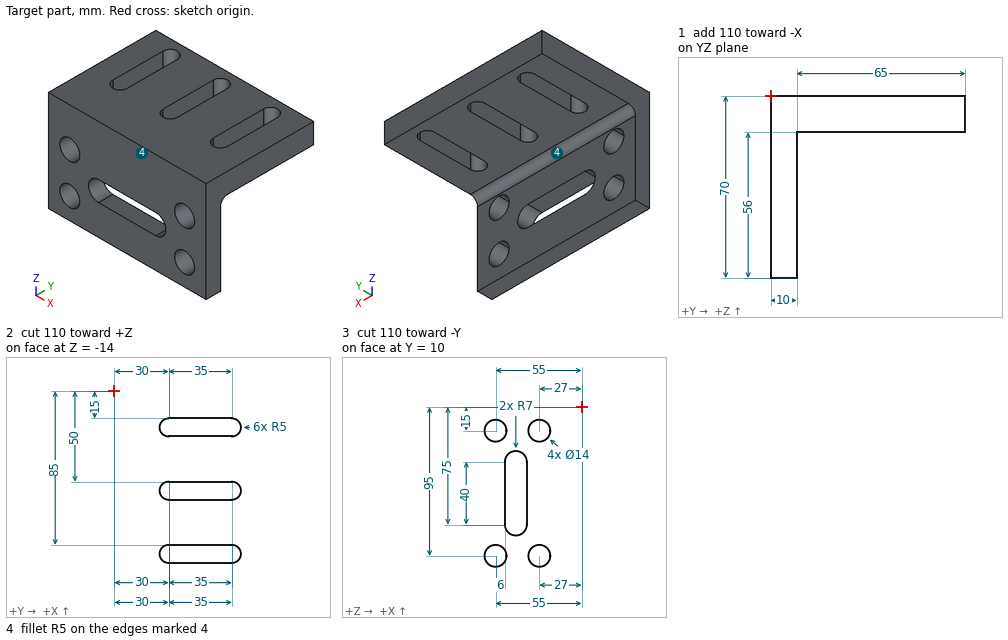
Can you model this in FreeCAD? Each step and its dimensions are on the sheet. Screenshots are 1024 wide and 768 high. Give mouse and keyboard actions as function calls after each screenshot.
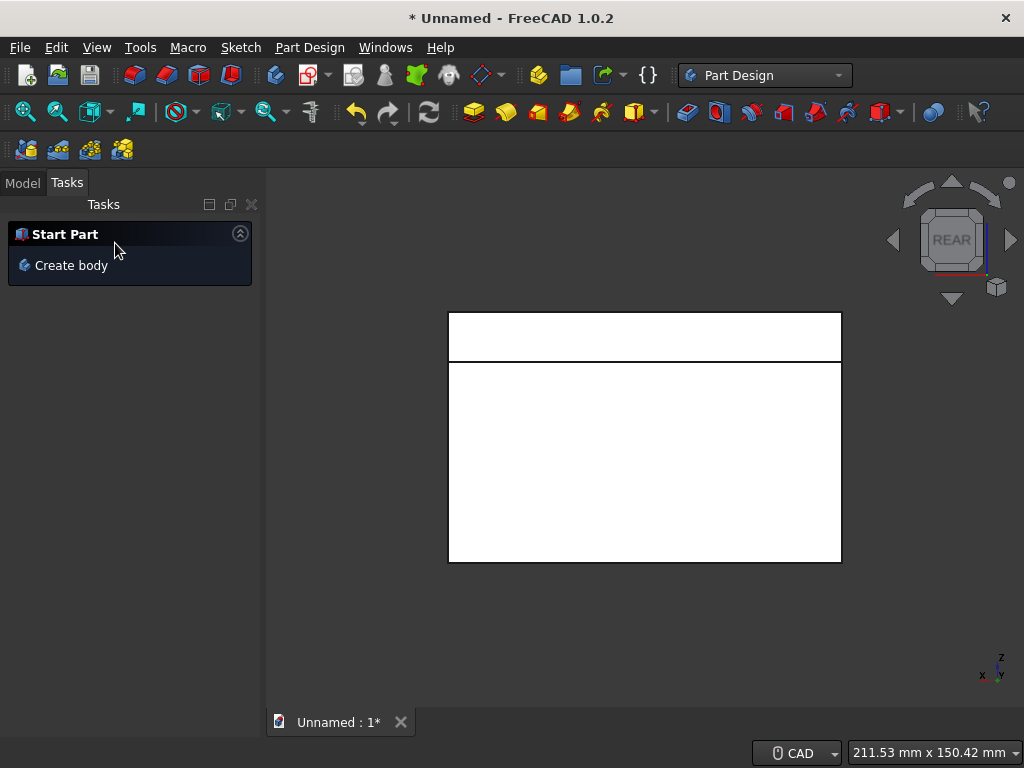
click(645, 462)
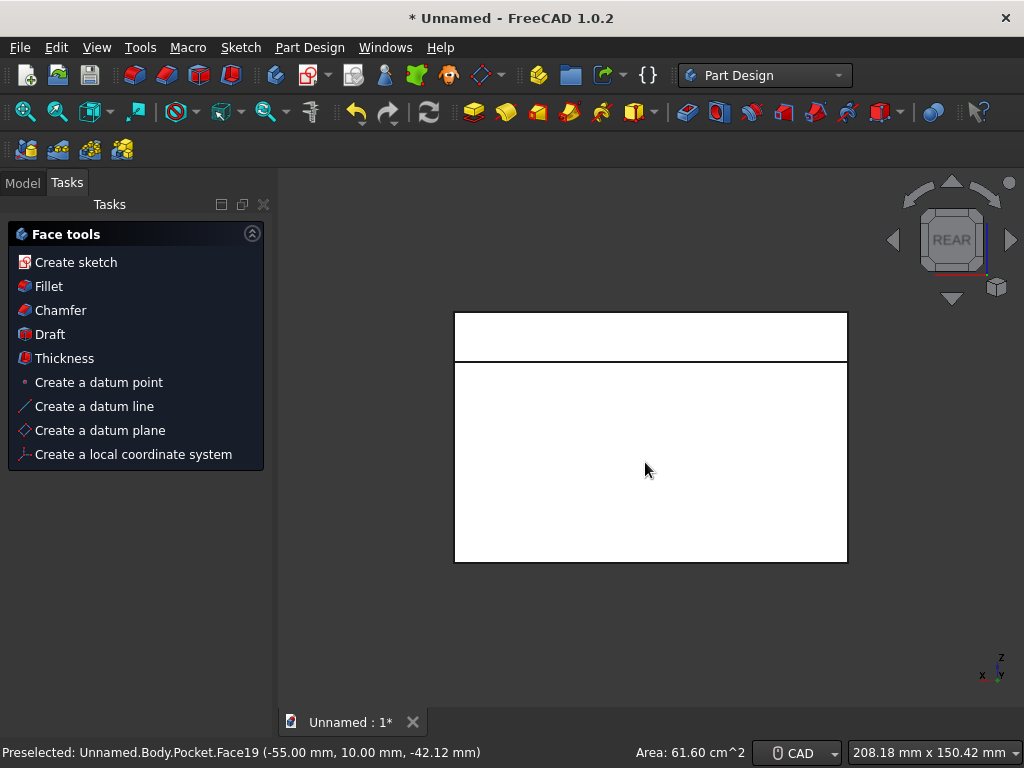
click(308, 76)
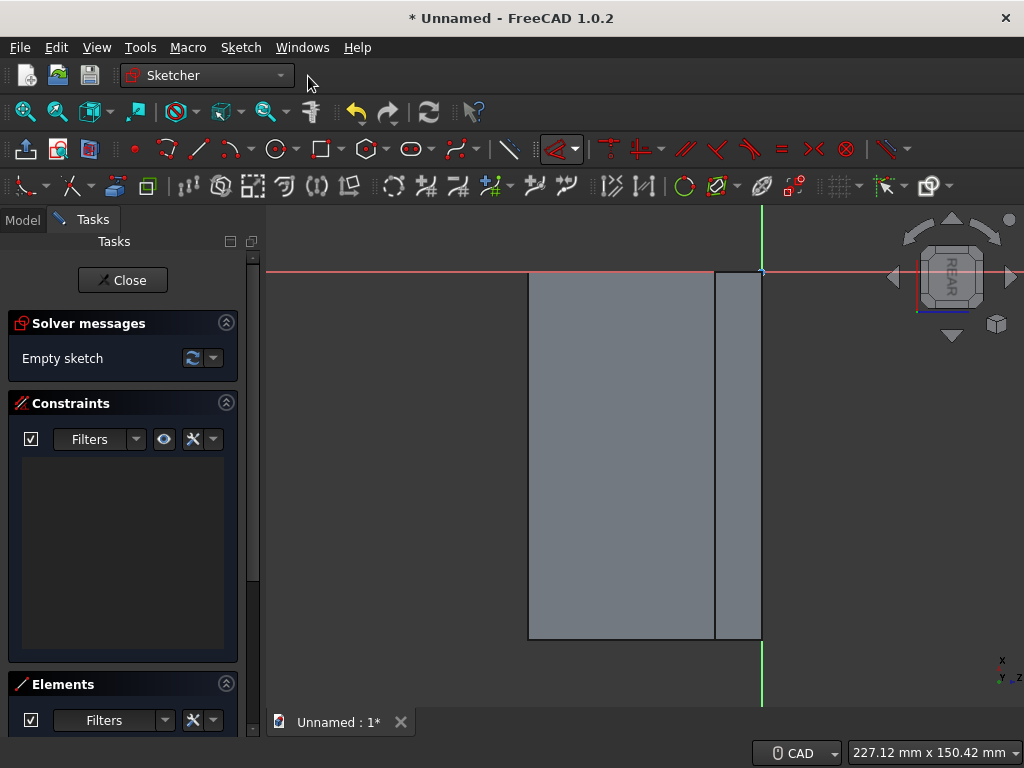
key(q)
key(s)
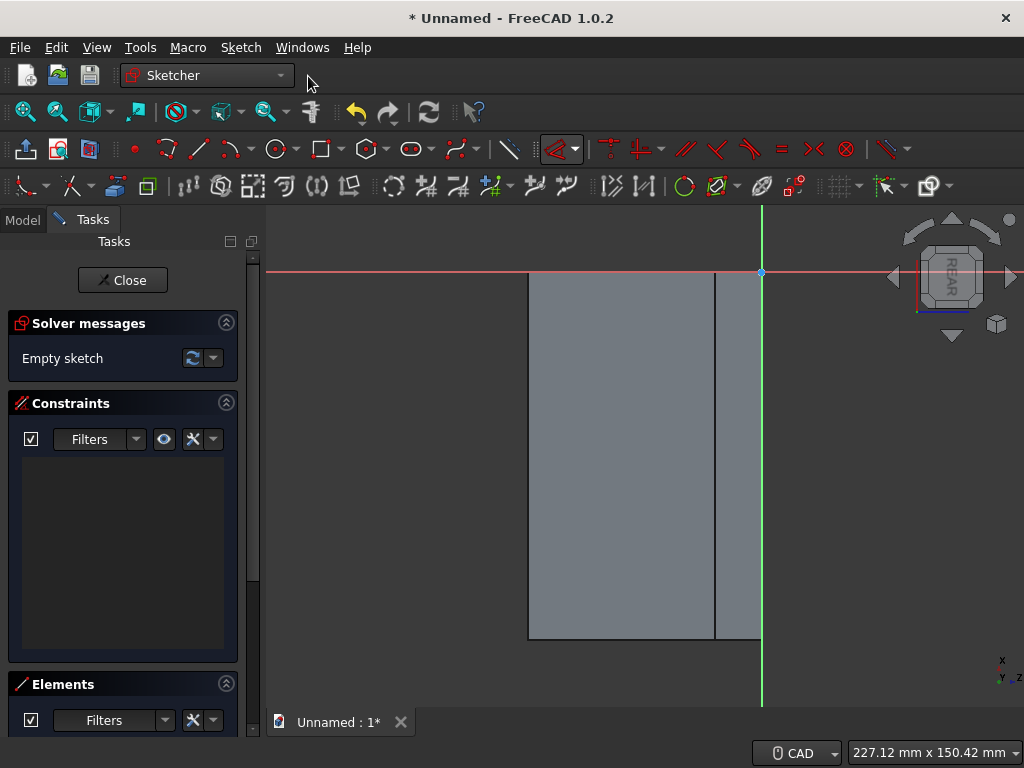
click(412, 150)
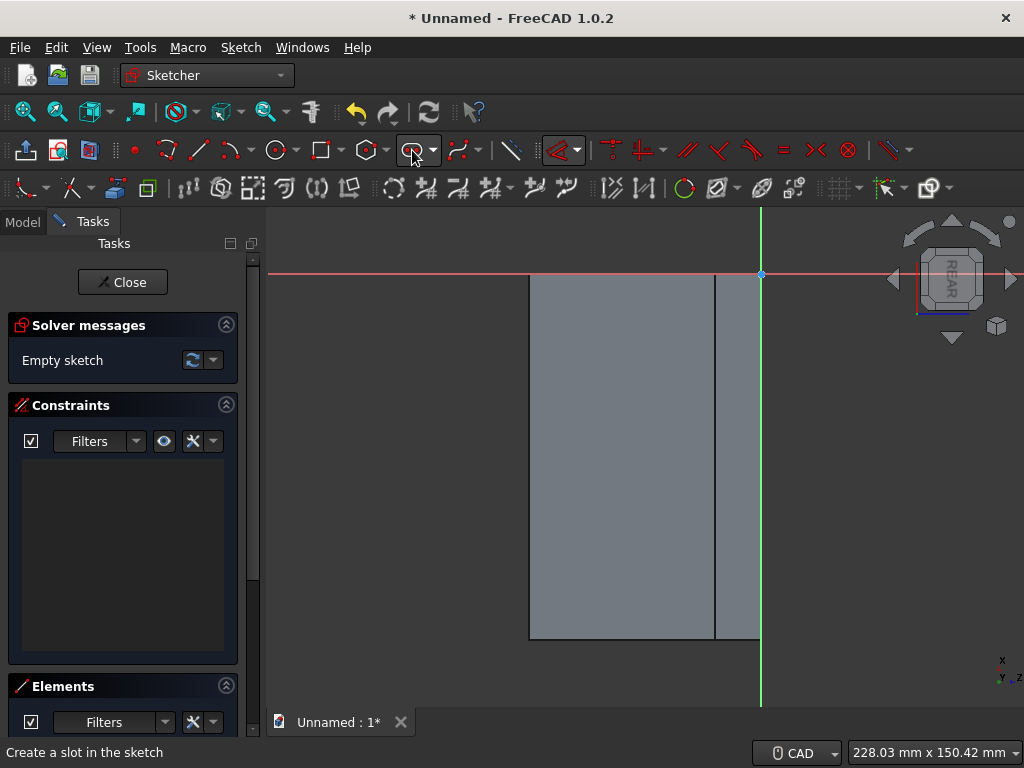
click(622, 523)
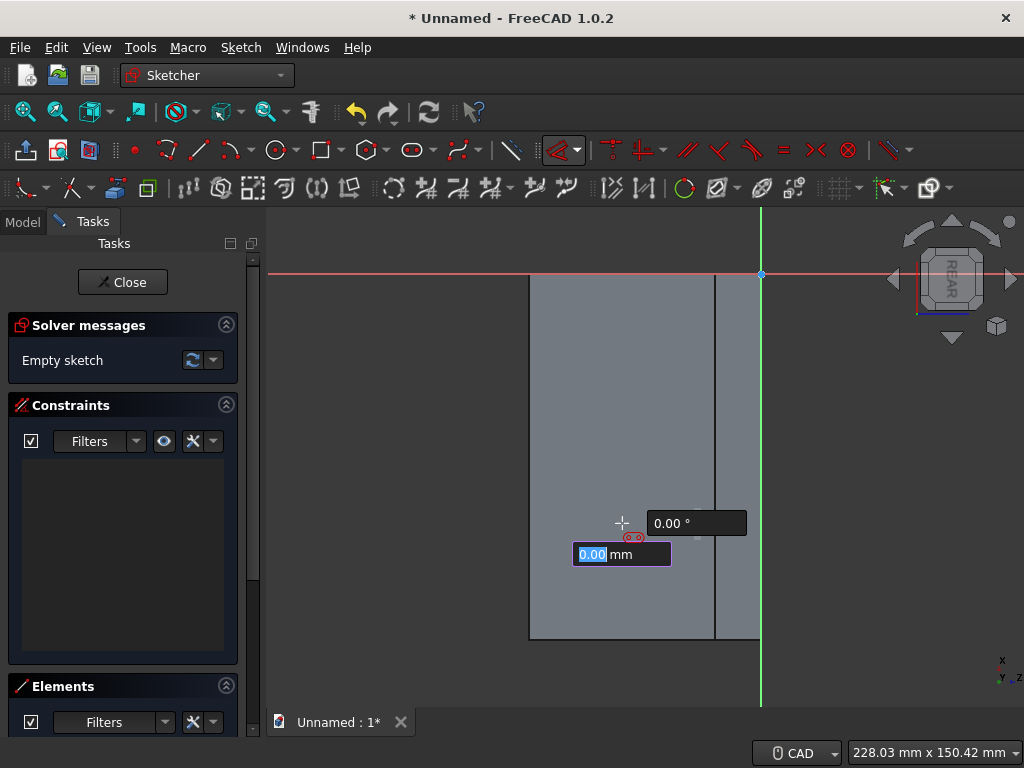
click(622, 391)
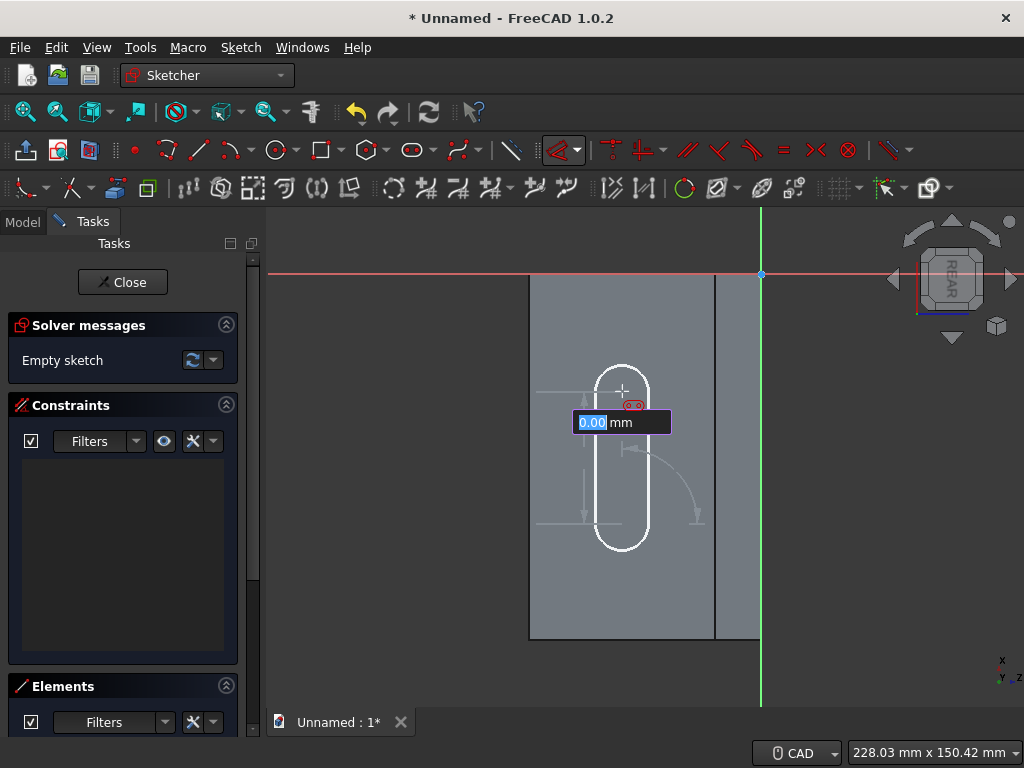
click(598, 457)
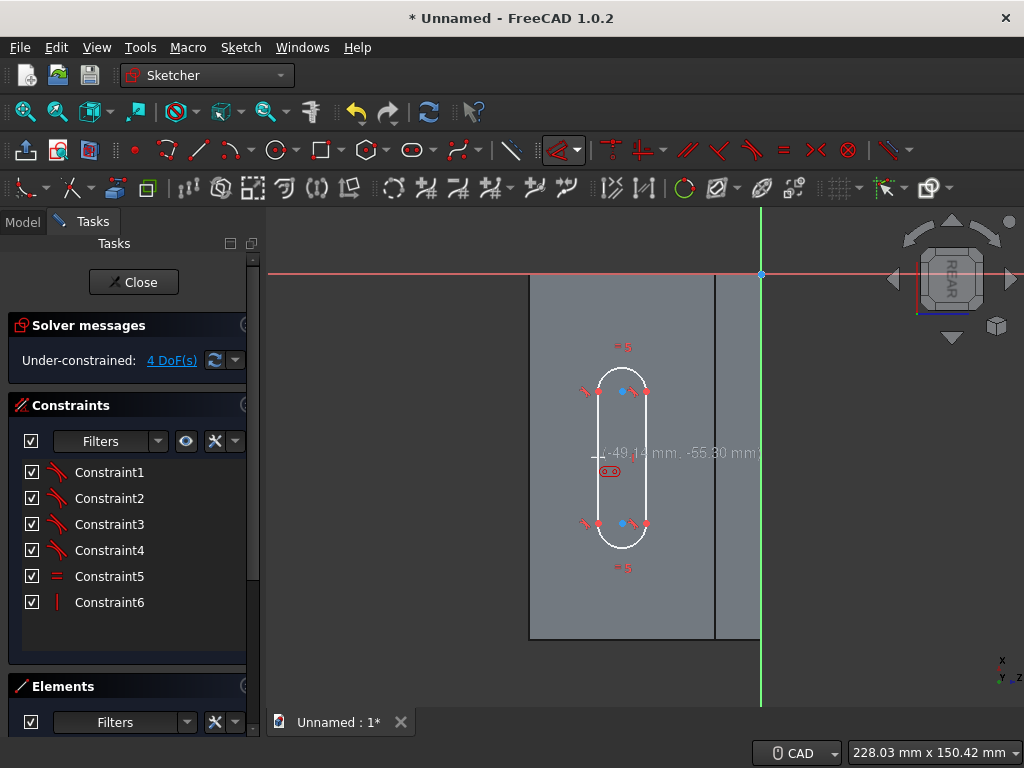
key(g)
key(c)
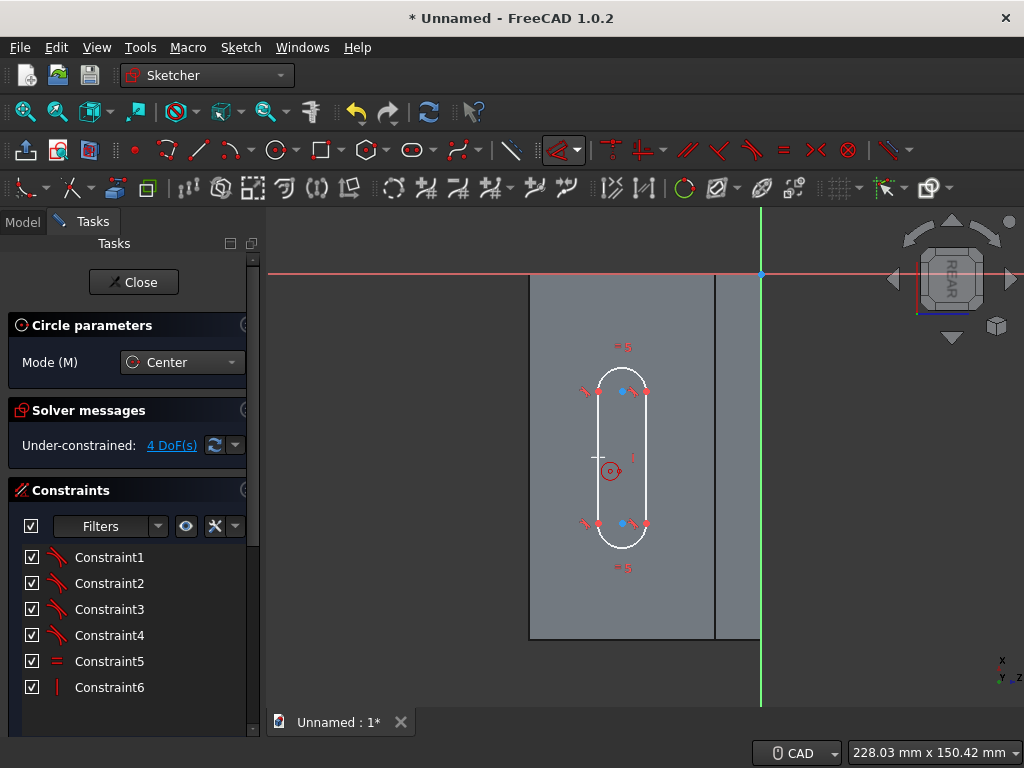
click(579, 590)
move(595, 574)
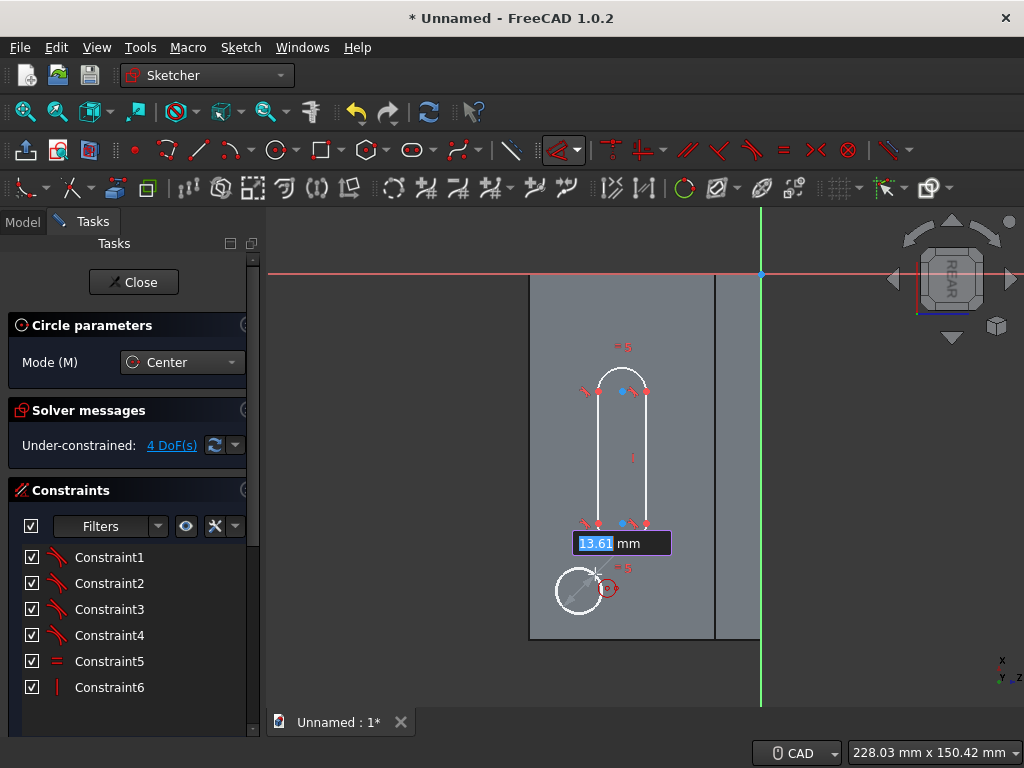
text(14)
key(Return)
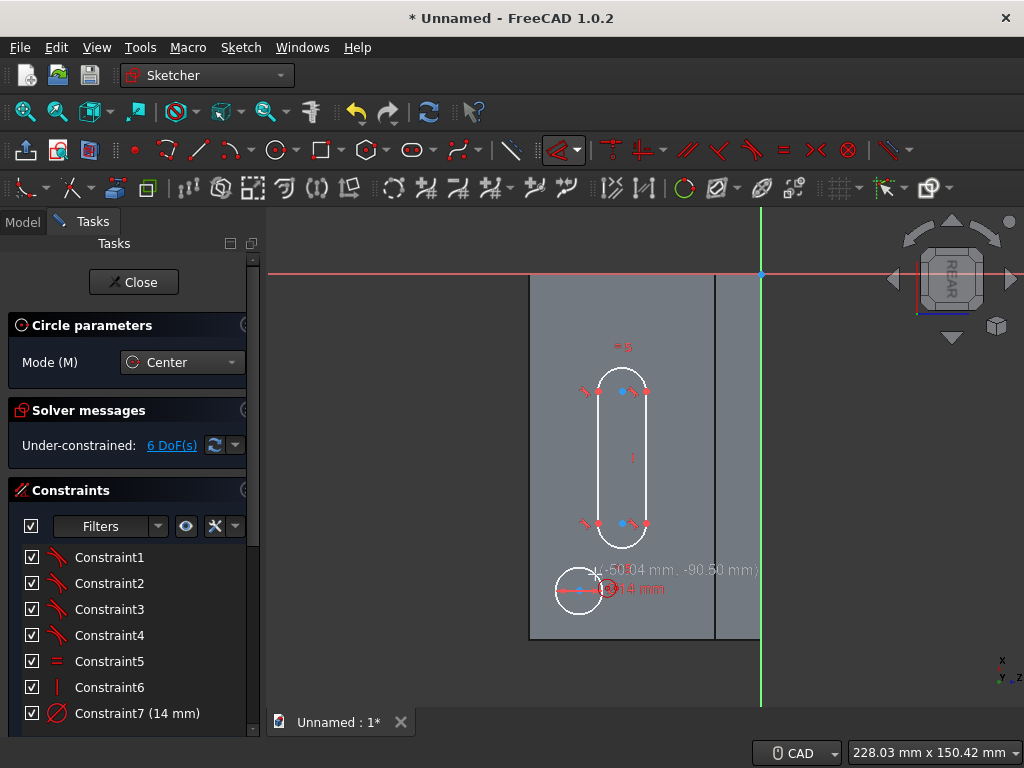
click(579, 324)
move(595, 308)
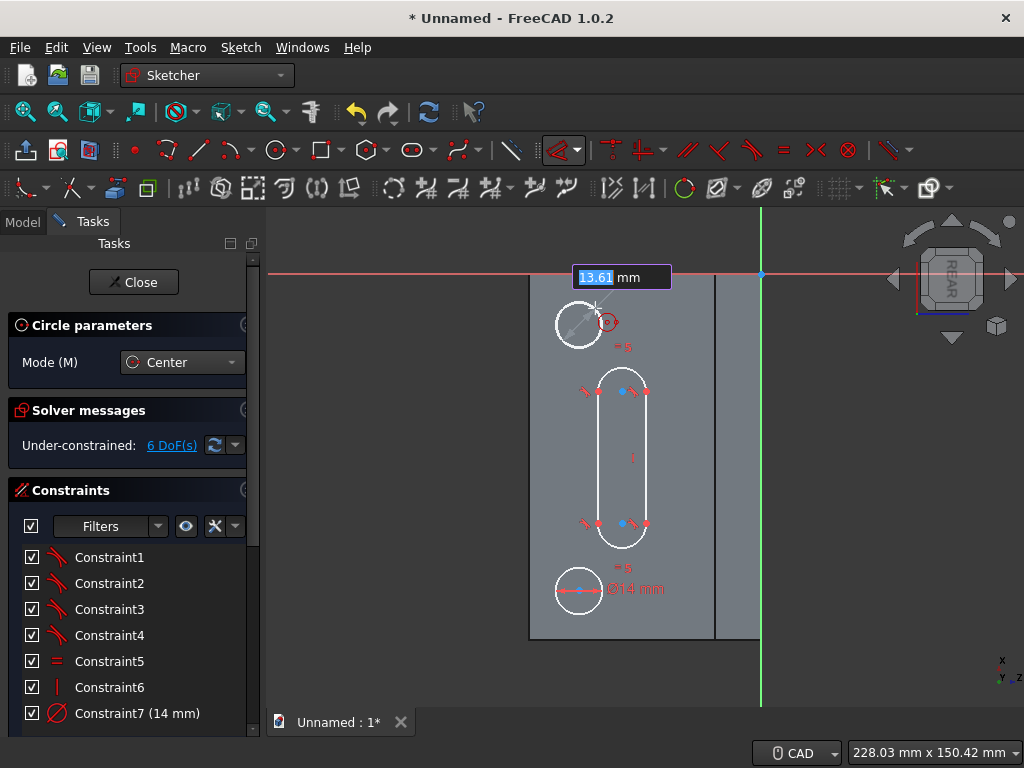
text(14)
key(Return)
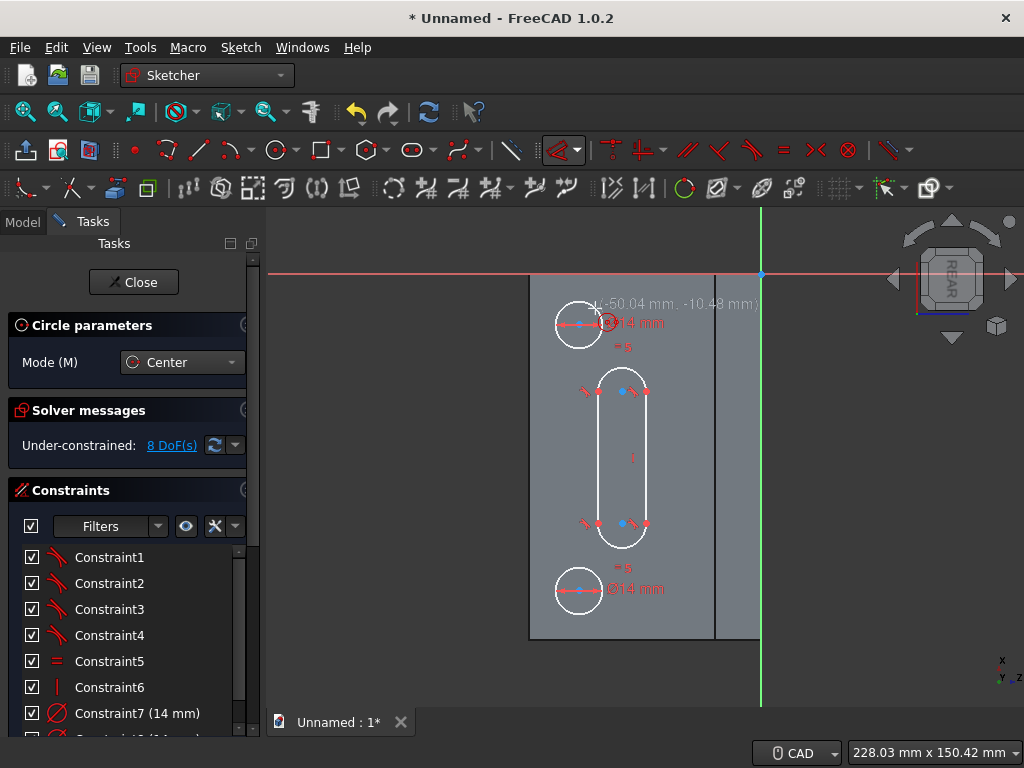
click(672, 324)
move(688, 308)